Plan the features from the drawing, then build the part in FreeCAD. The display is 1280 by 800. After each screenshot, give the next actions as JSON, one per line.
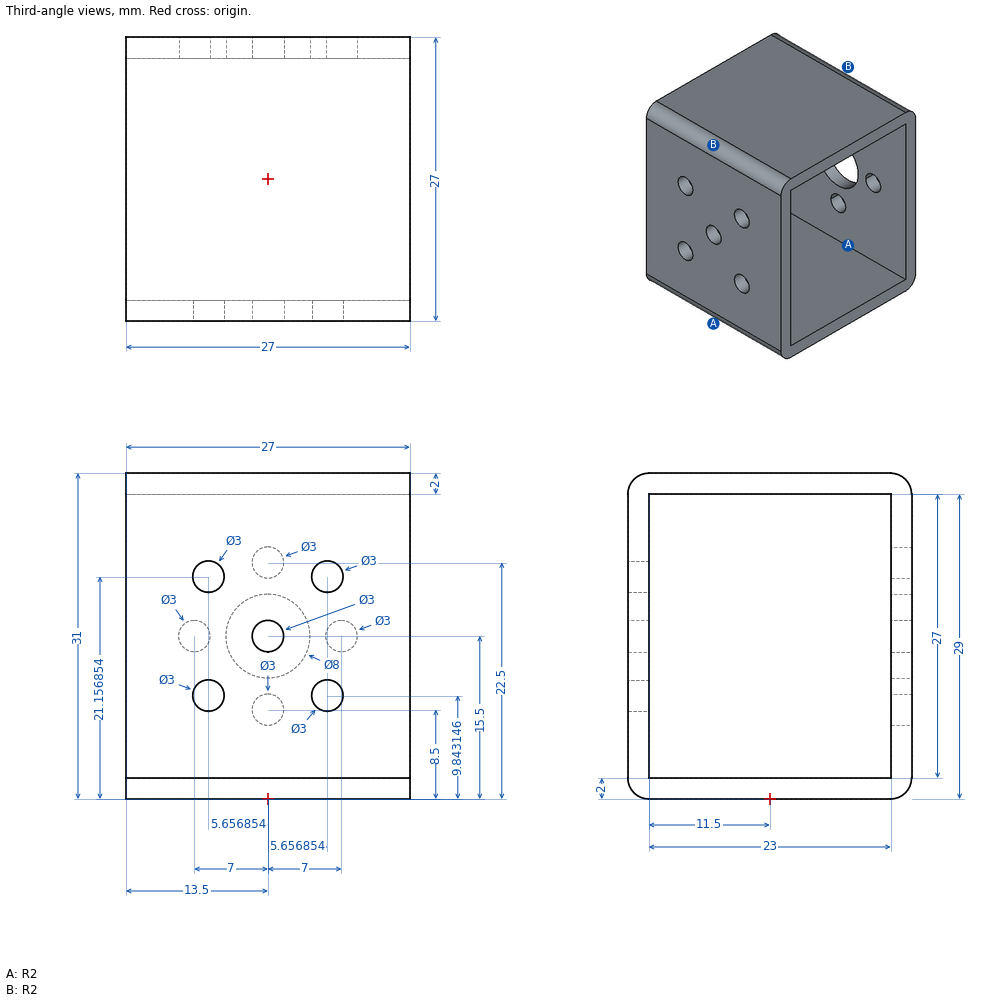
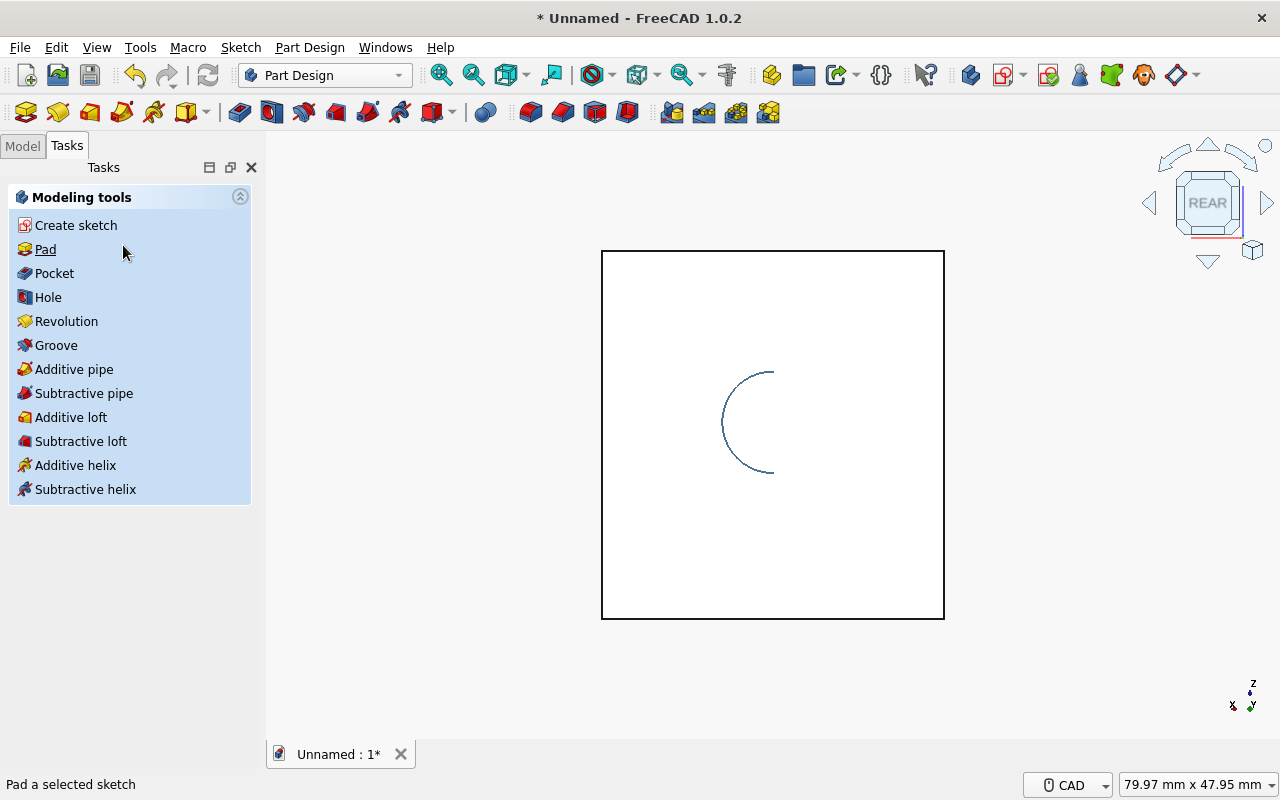
{"action": "left_click", "coordinate": [240, 112]}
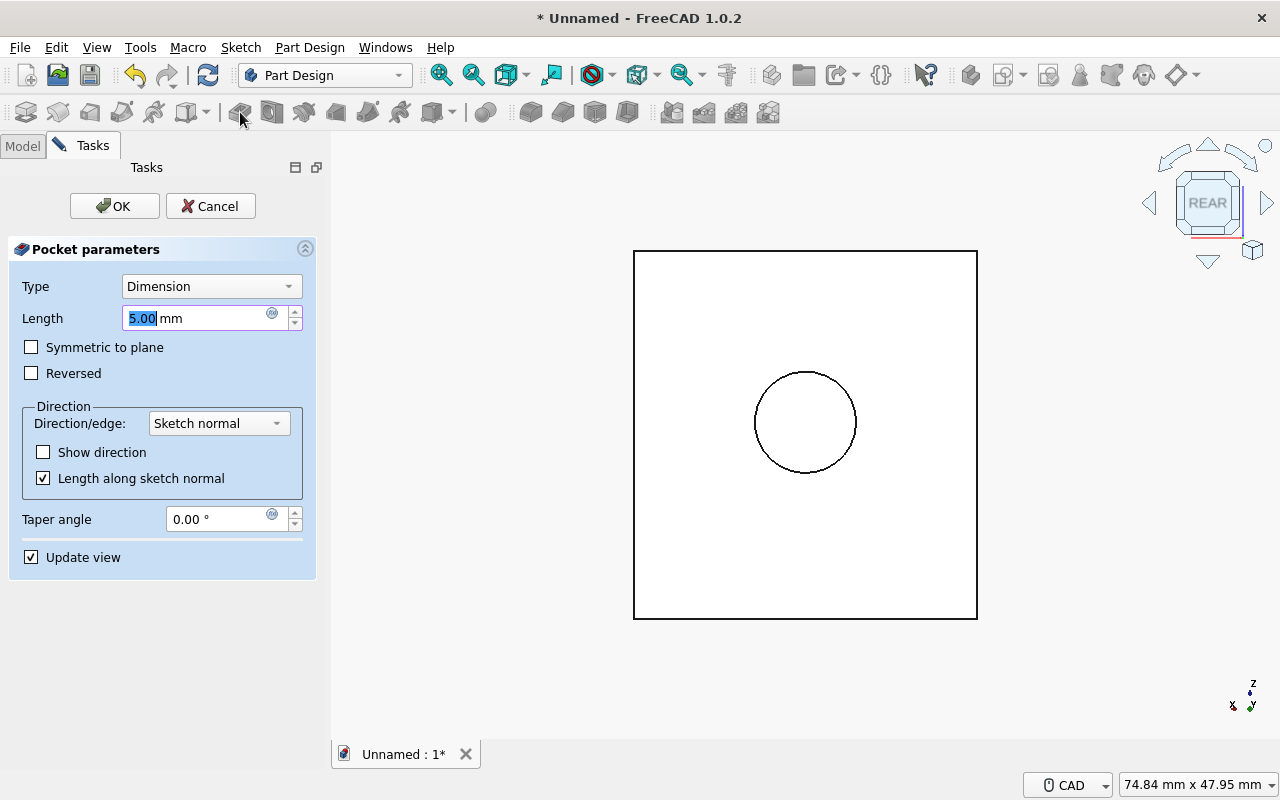
{"action": "left_click", "coordinate": [212, 286]}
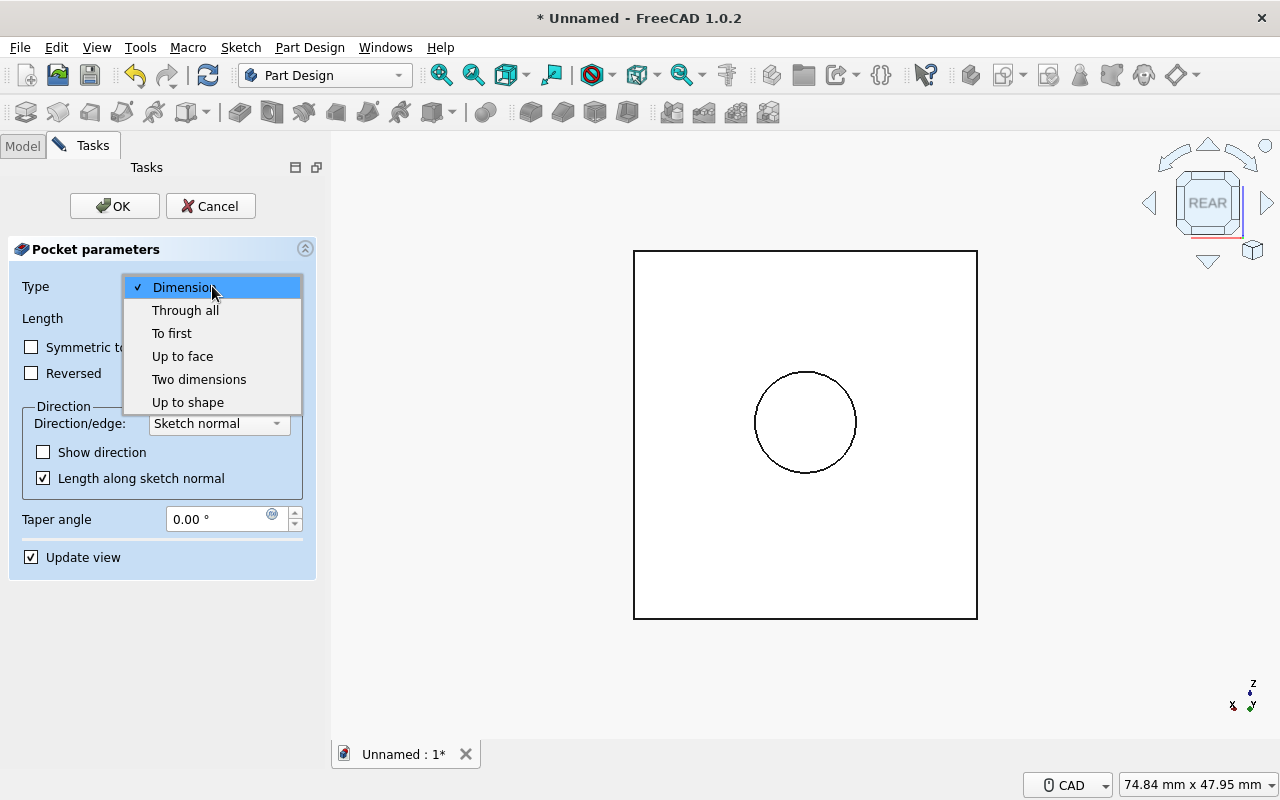
{"action": "left_click", "coordinate": [212, 334]}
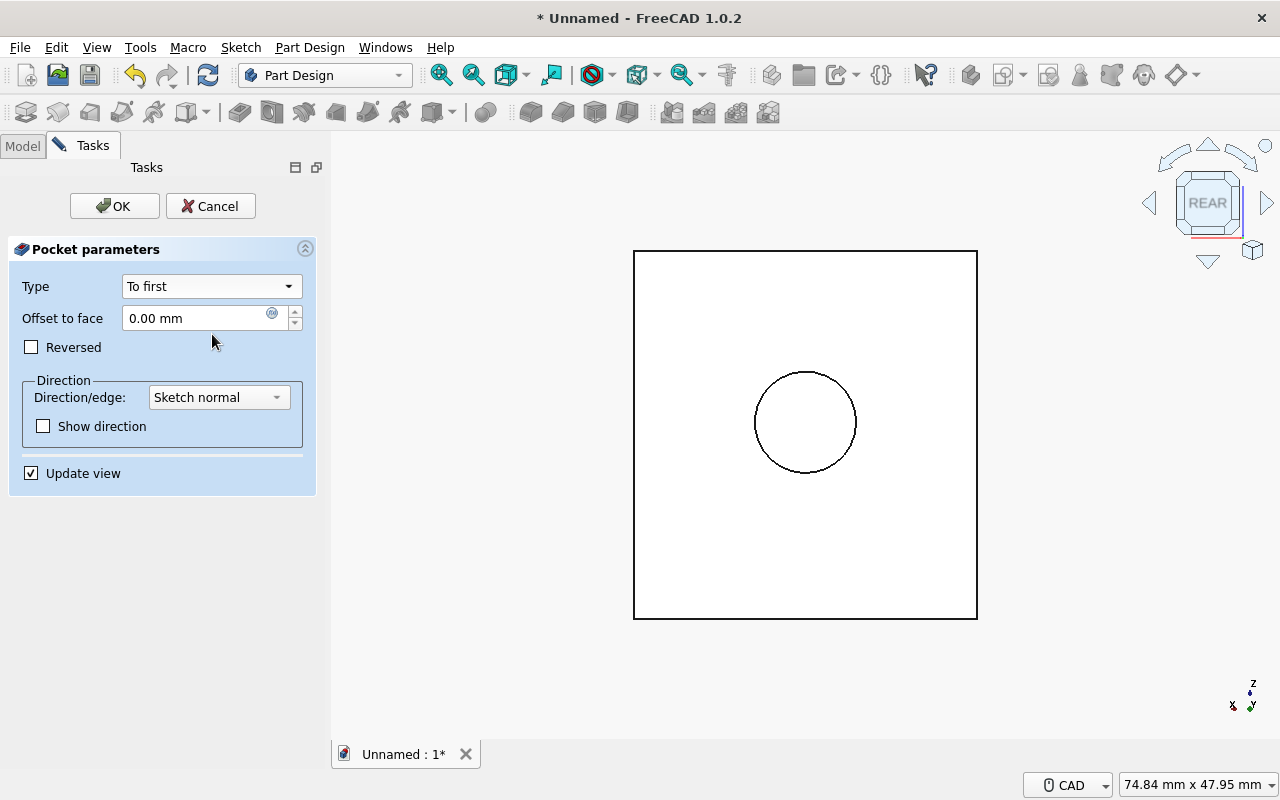
{"action": "left_click", "coordinate": [115, 206]}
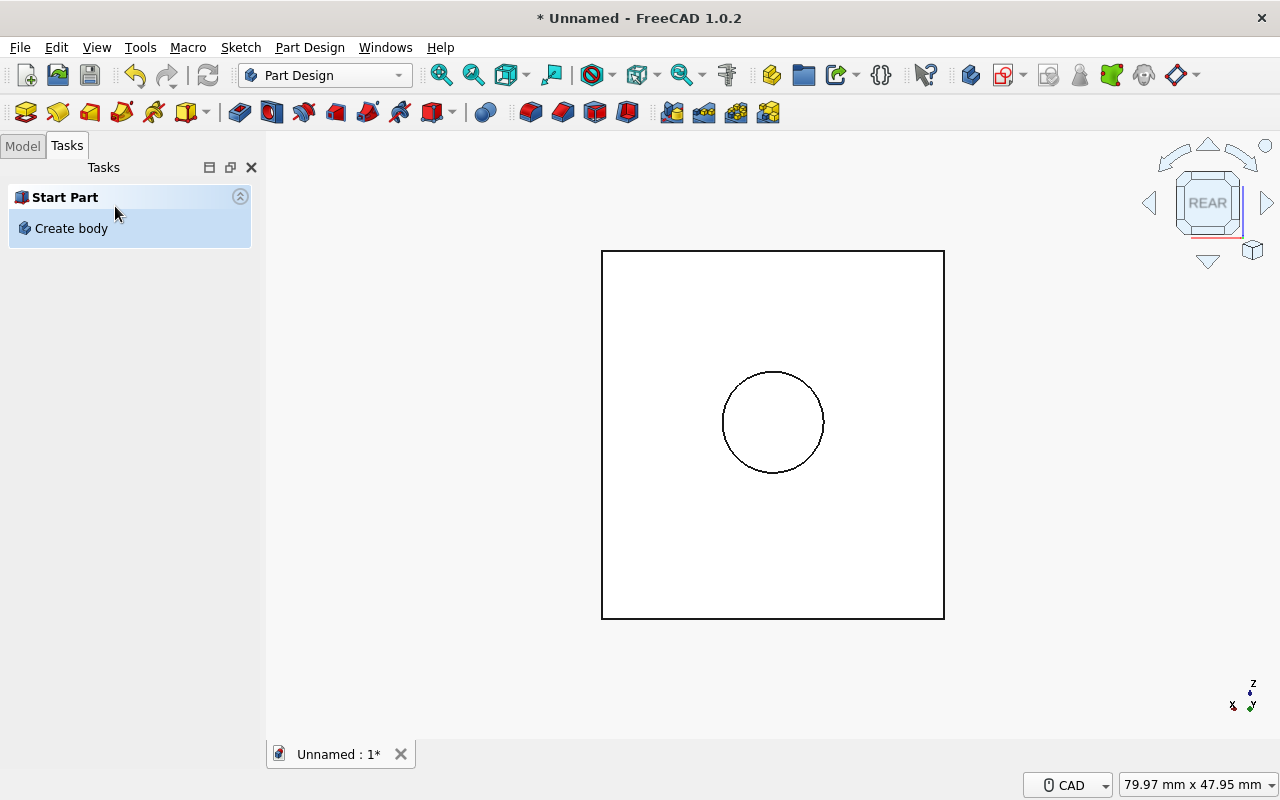
{"action": "left_click", "coordinate": [822, 539]}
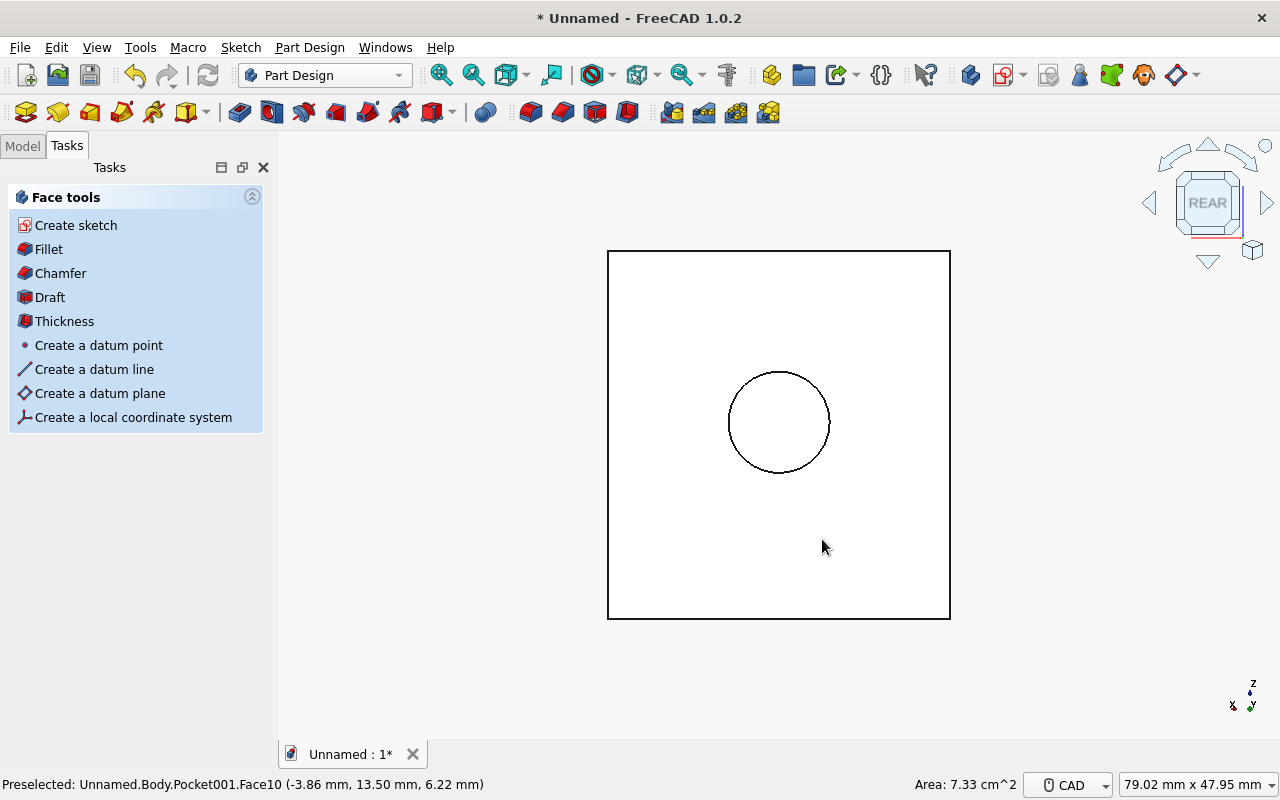
{"action": "left_click", "coordinate": [1004, 76]}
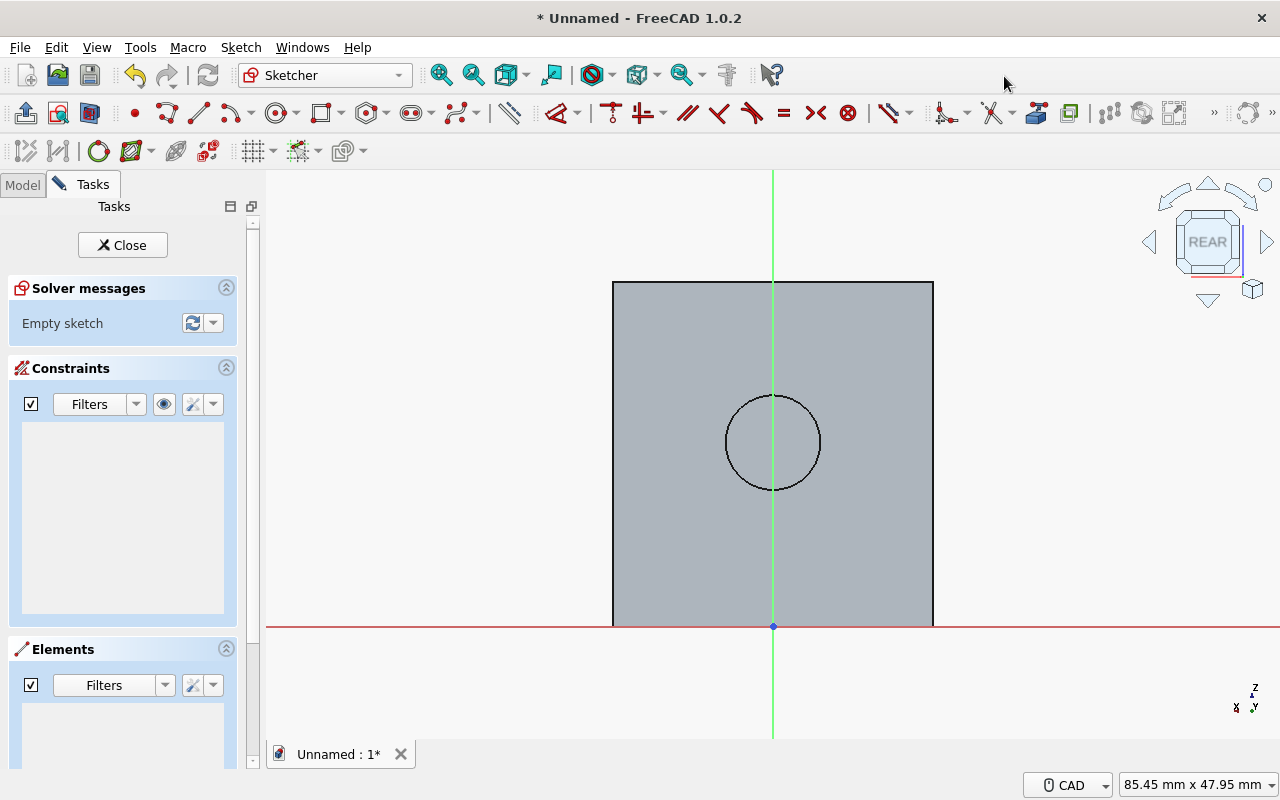
{"action": "scroll", "coordinate": [780, 533], "scroll_direction": "up", "scroll_amount": 12}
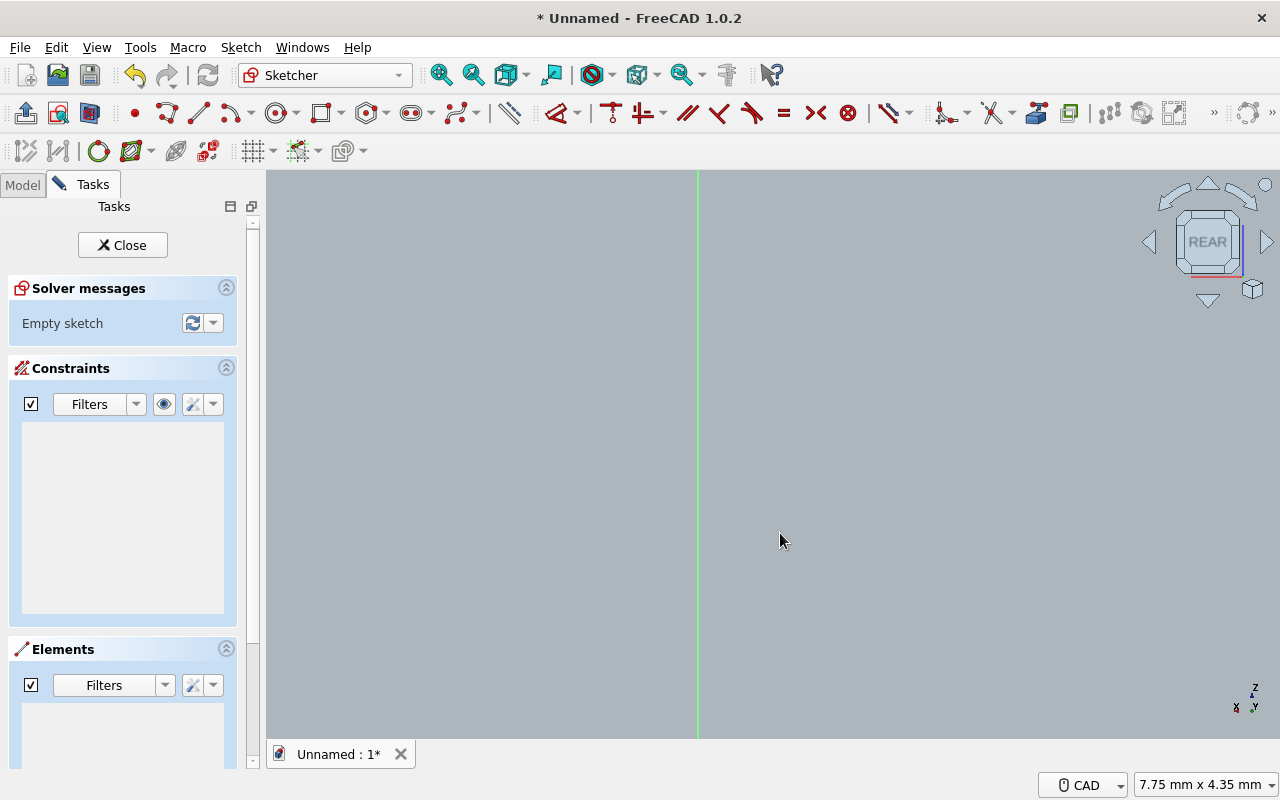
{"action": "left_click", "coordinate": [276, 114]}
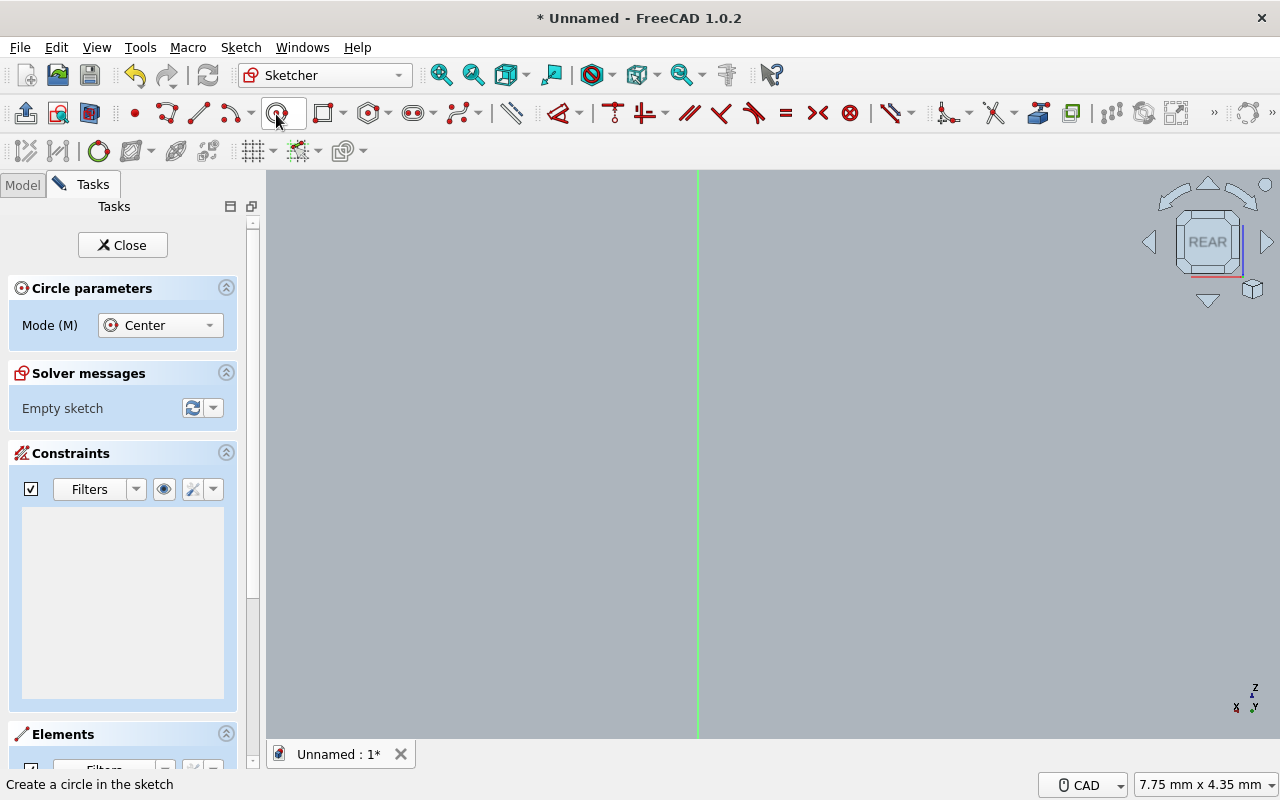
{"action": "left_click", "coordinate": [698, 446]}
{"action": "mouse_move", "coordinate": [837, 307]}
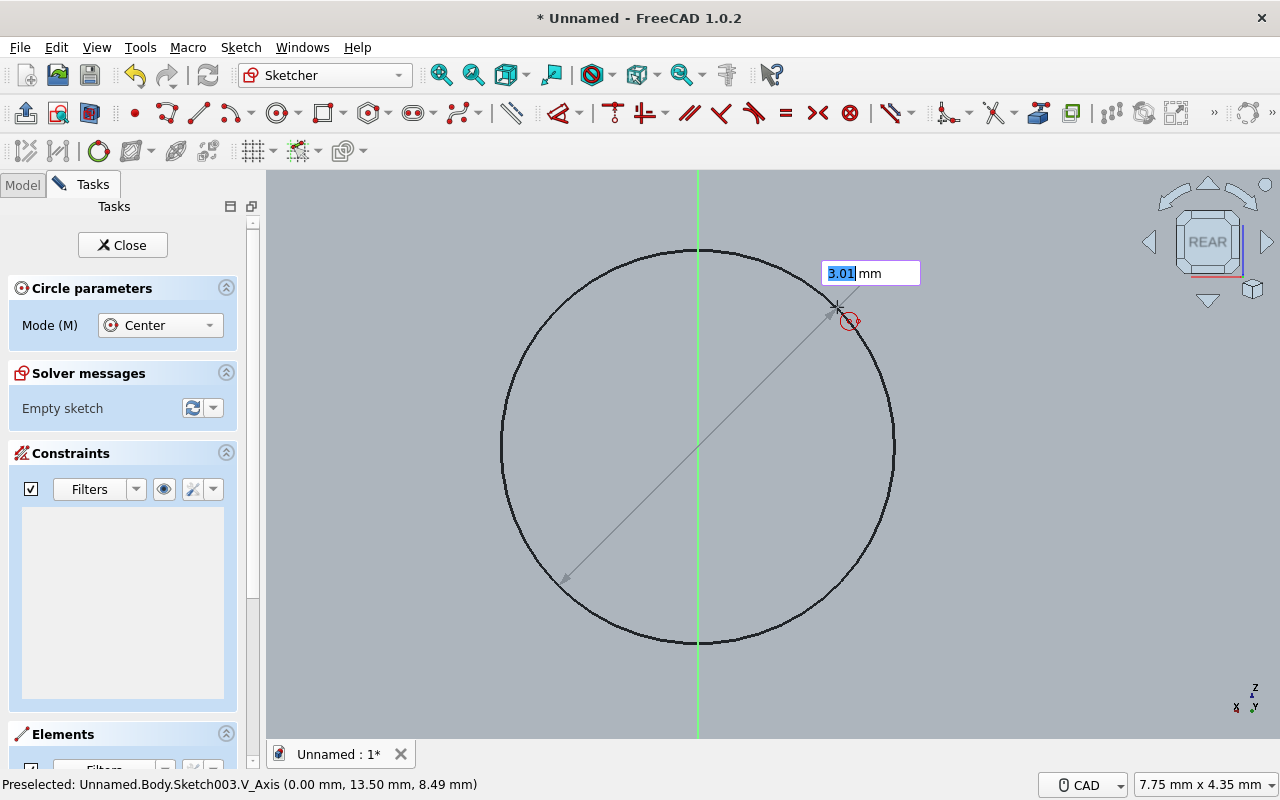
{"action": "type", "text": "3"}
{"action": "key", "text": "Return"}
{"action": "key", "text": "Escape"}